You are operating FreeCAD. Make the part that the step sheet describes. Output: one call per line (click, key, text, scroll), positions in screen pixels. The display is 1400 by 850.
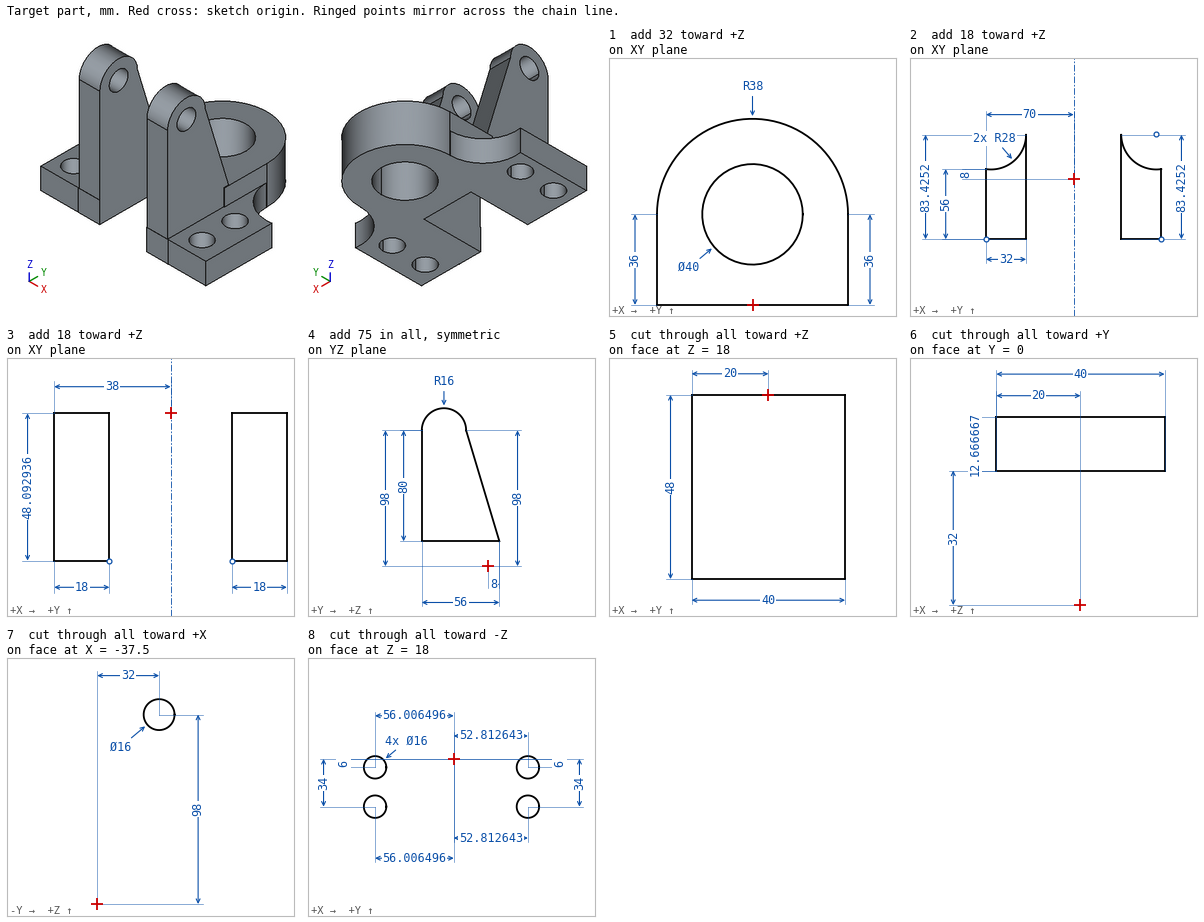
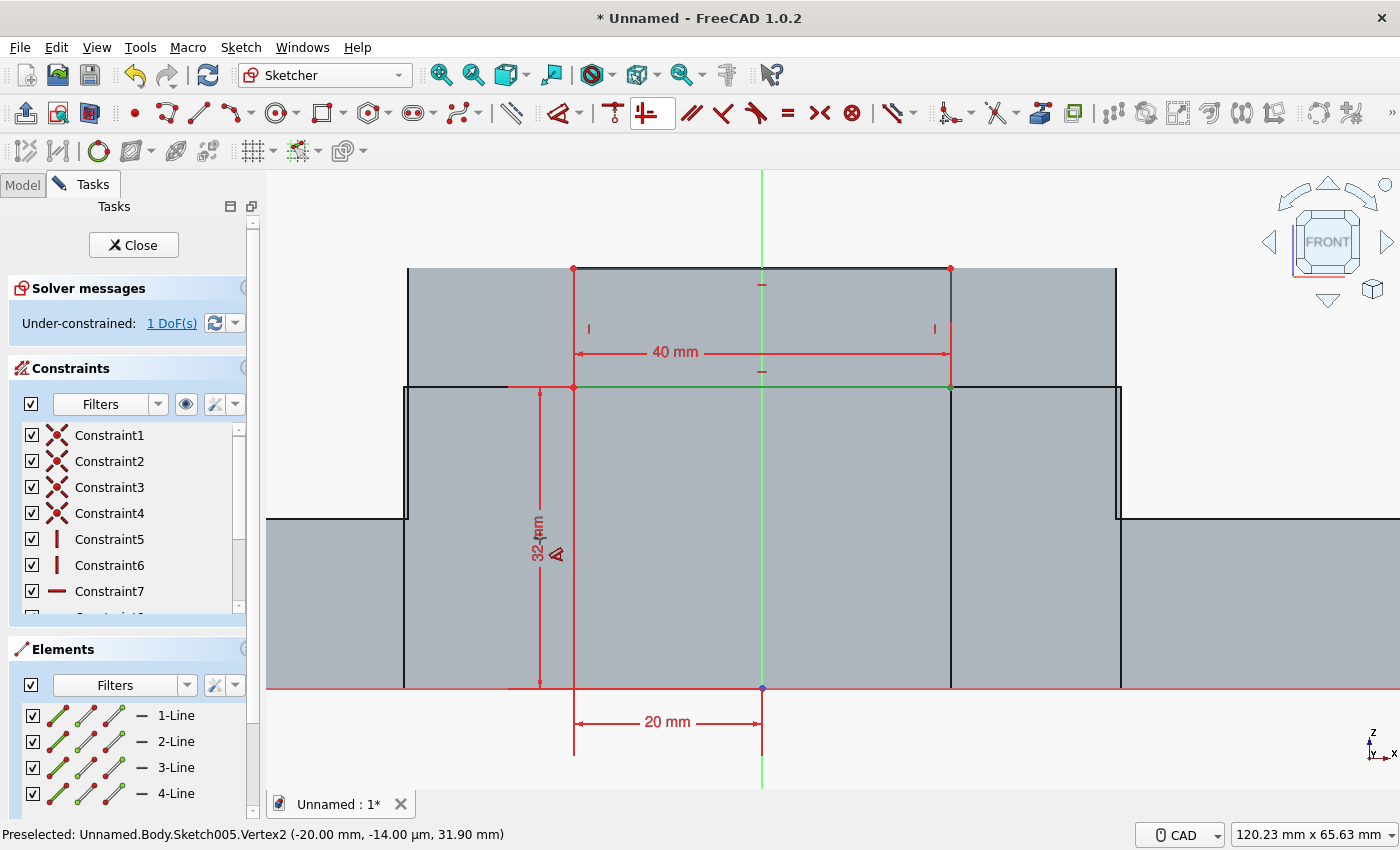
click(574, 304)
click(540, 328)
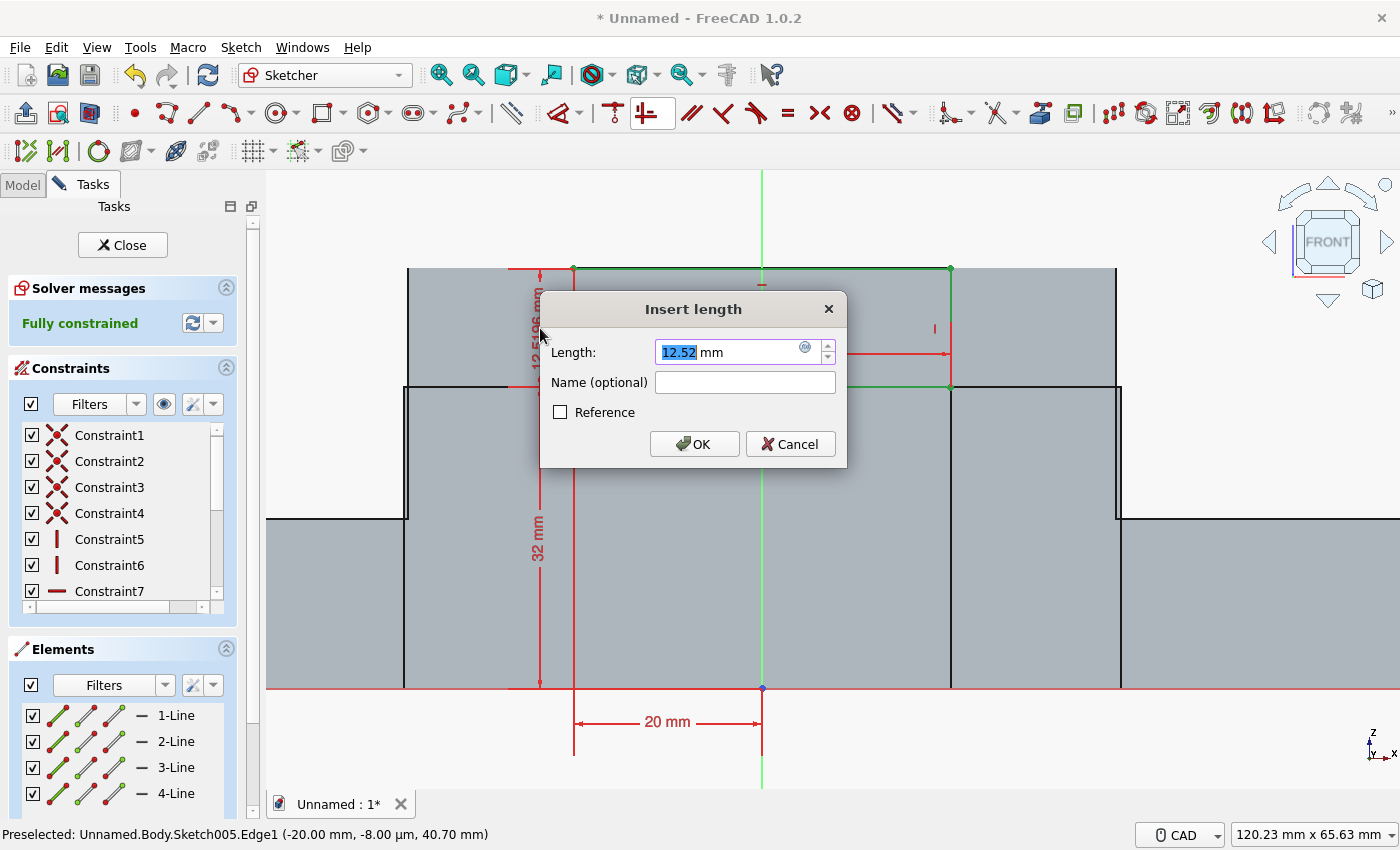
text(12.666667)
key(Return)
key(Escape)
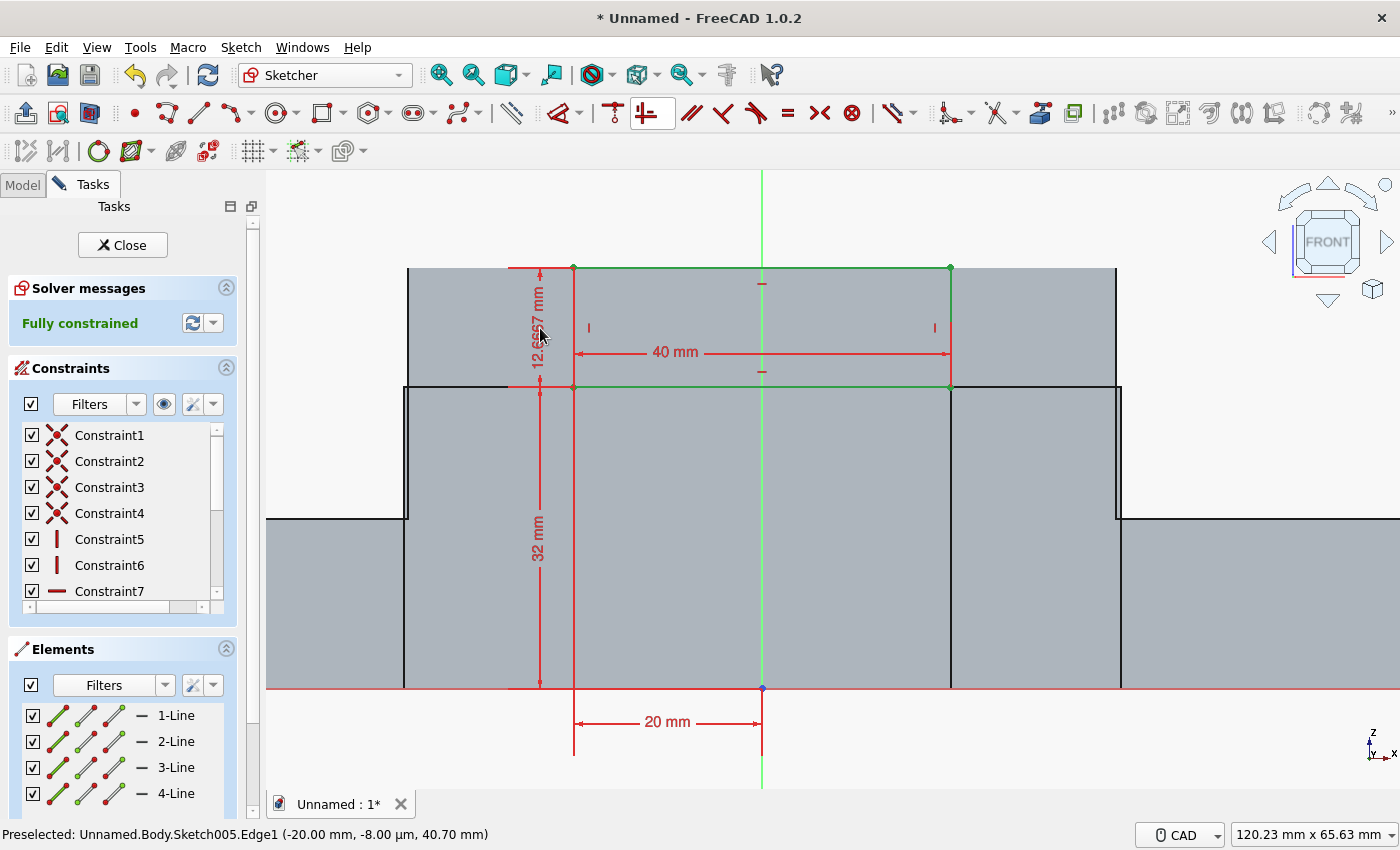
click(123, 245)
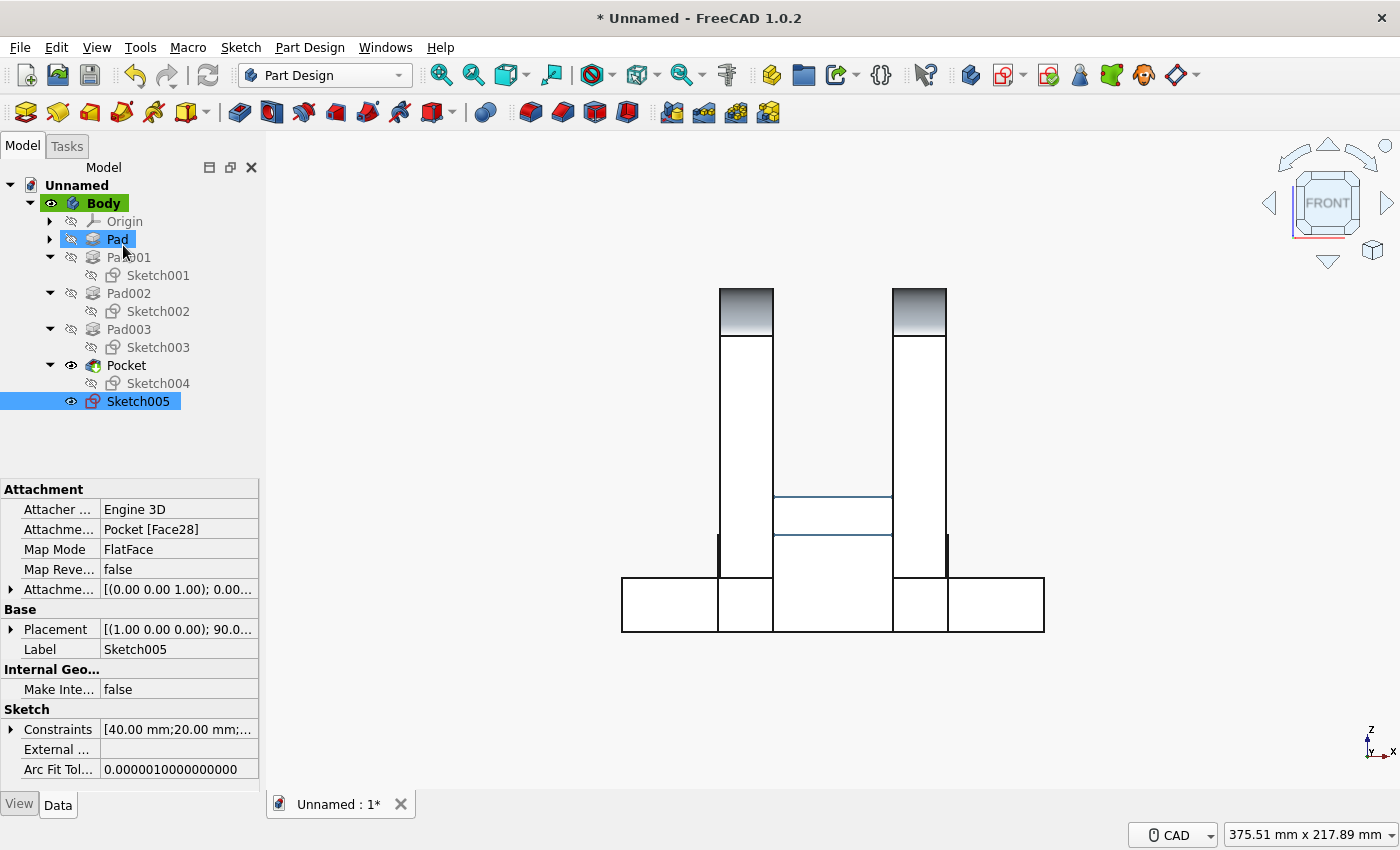
click(240, 112)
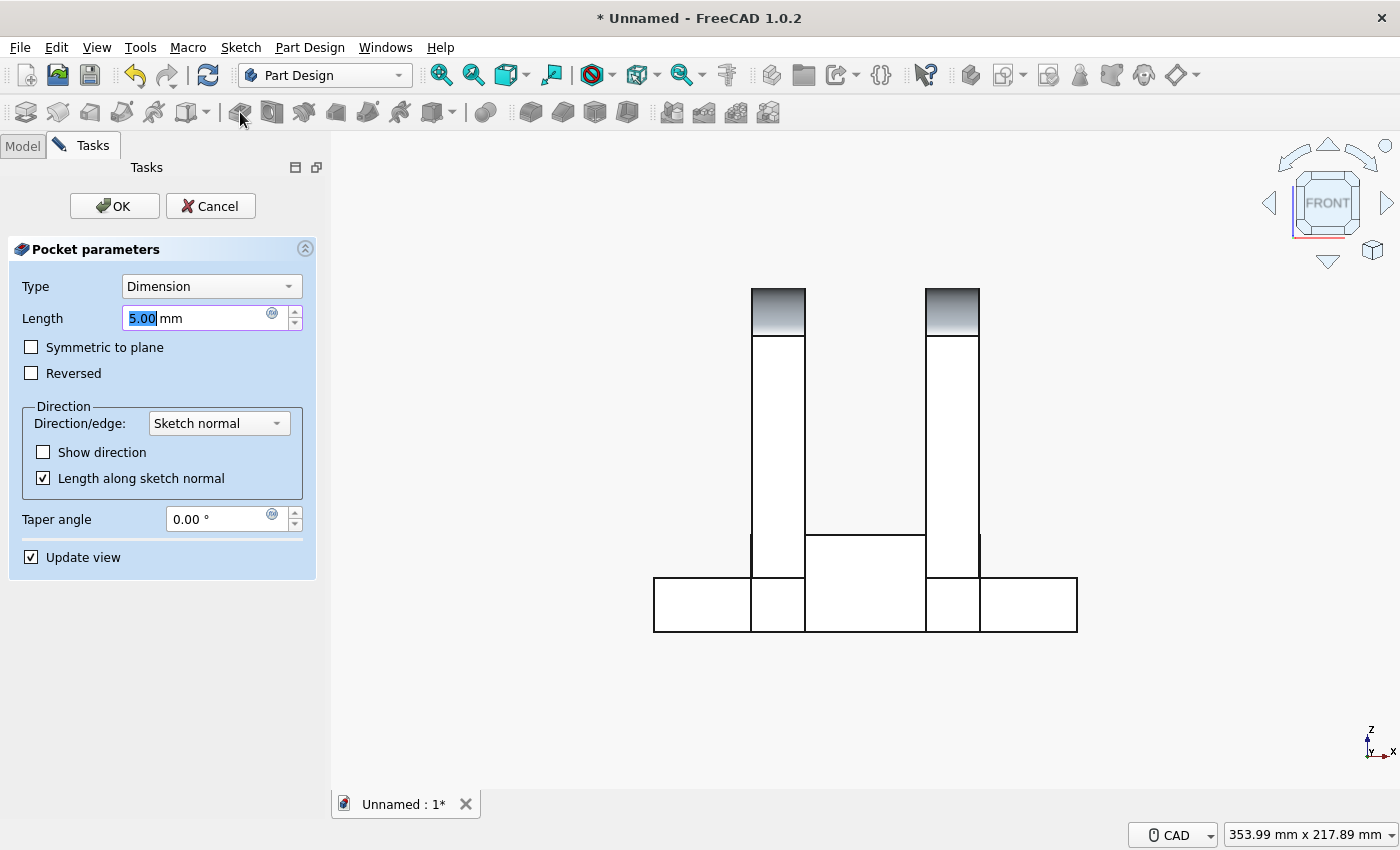
click(212, 286)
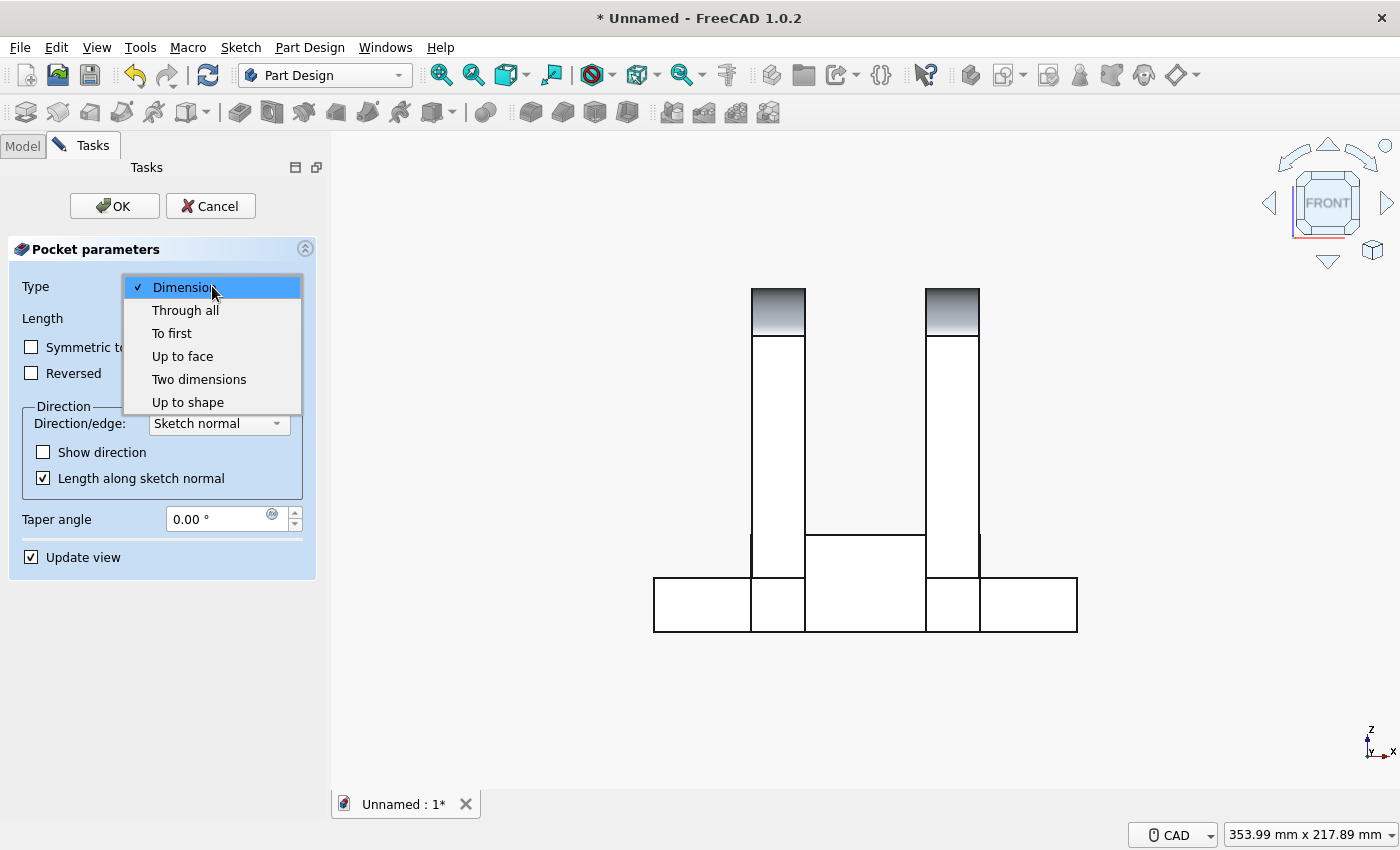
click(212, 310)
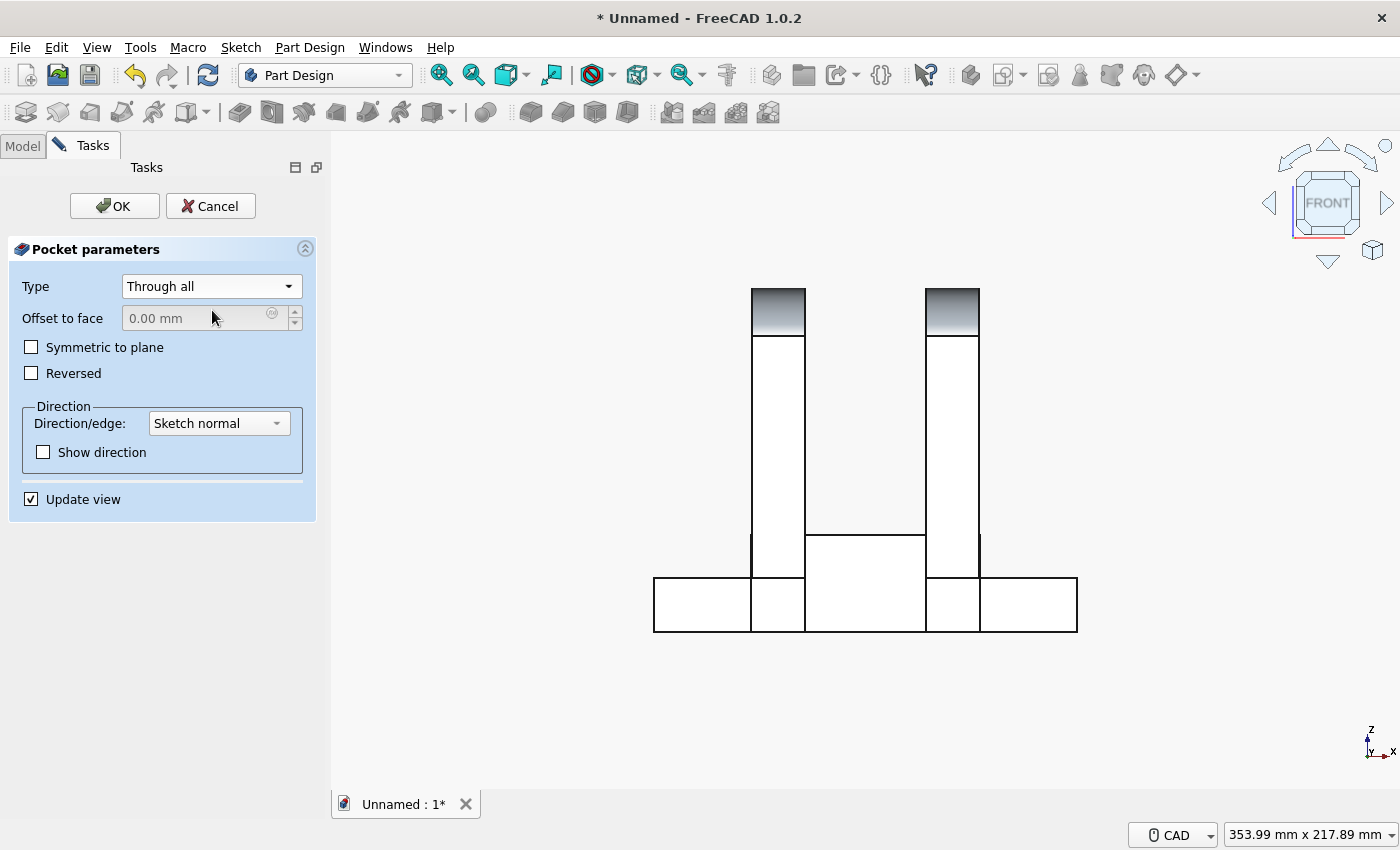
click(115, 206)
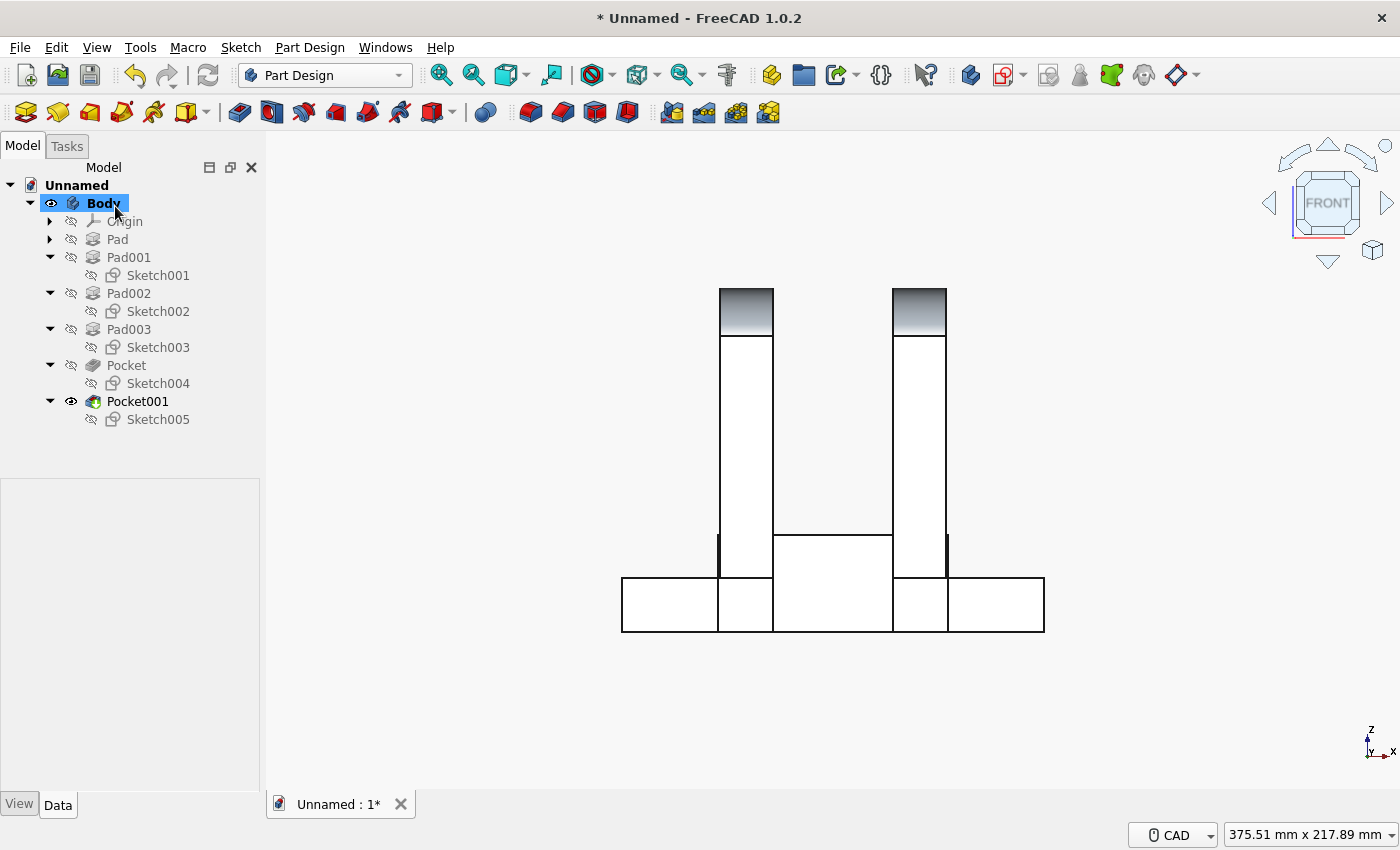
key(6)